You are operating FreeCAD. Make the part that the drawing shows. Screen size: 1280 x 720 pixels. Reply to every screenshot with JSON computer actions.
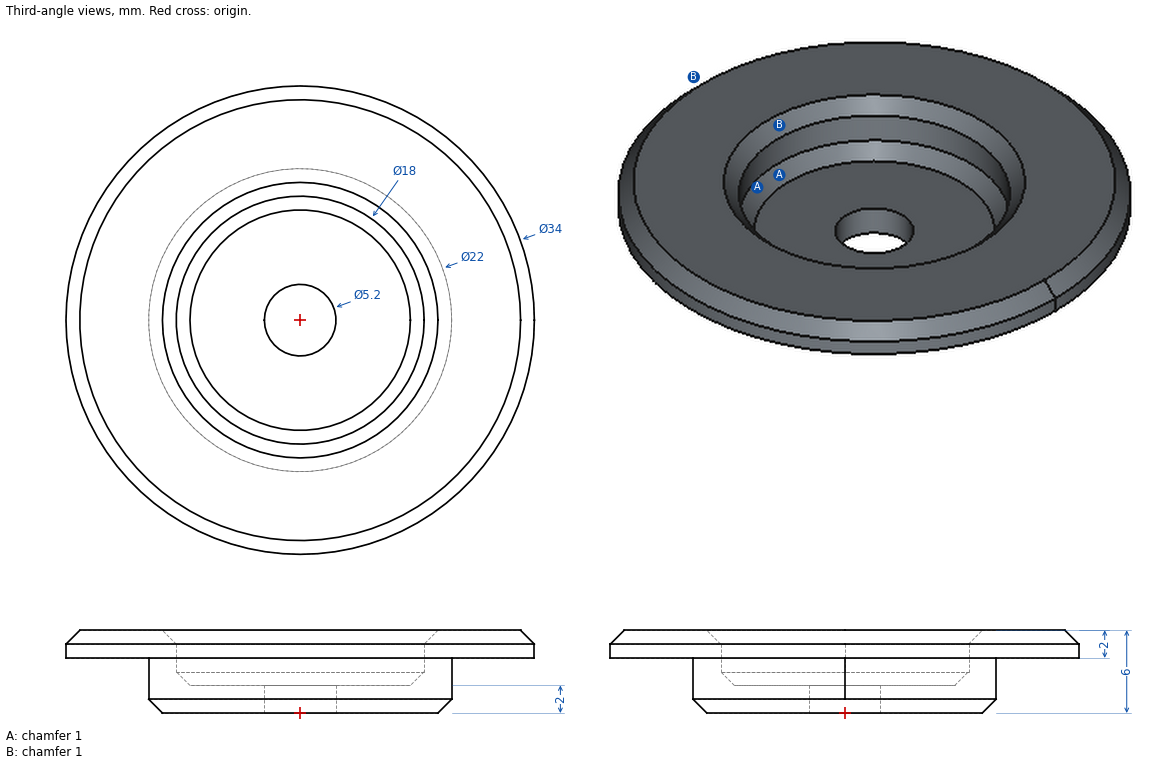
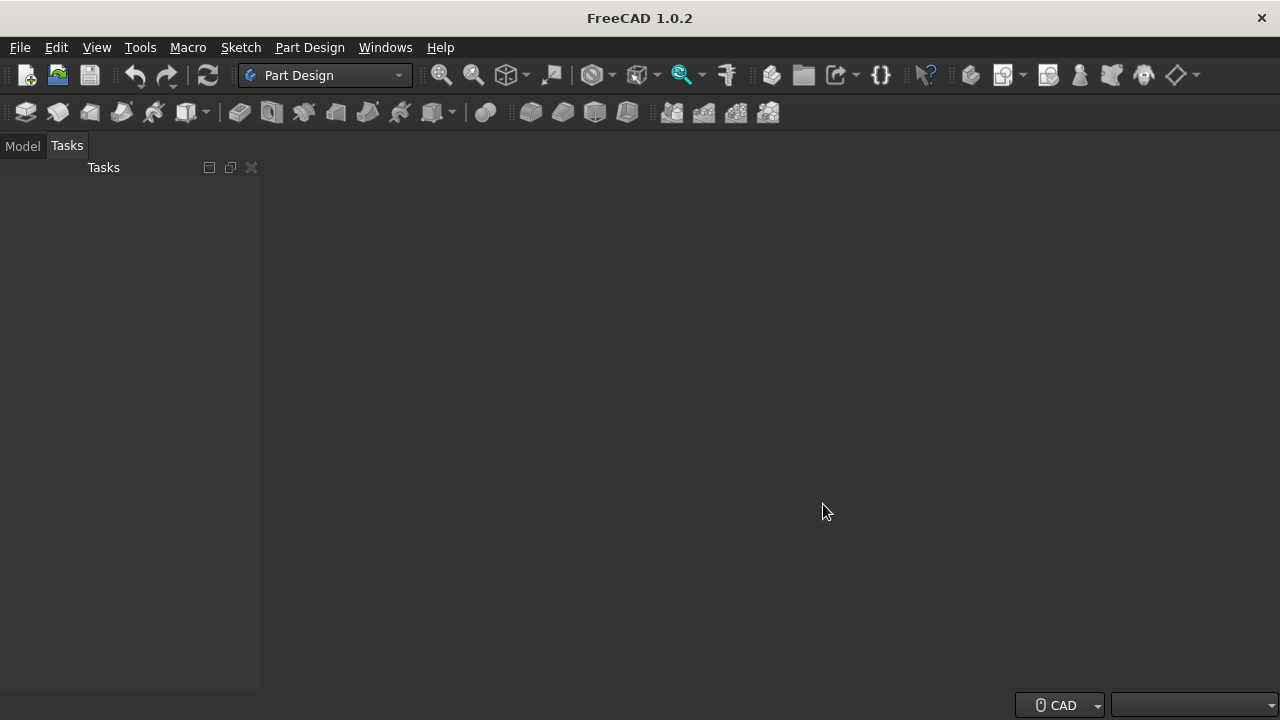
{"action": "left_click", "coordinate": [26, 76]}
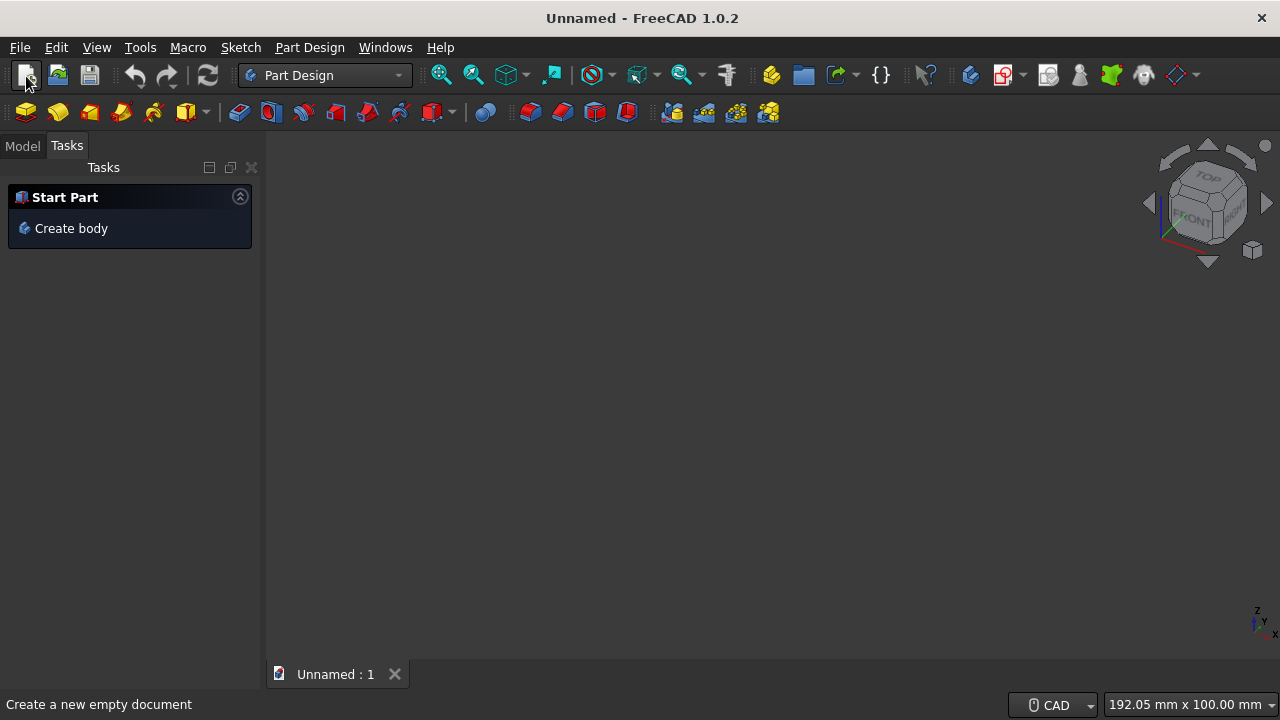
{"action": "left_click", "coordinate": [1004, 76]}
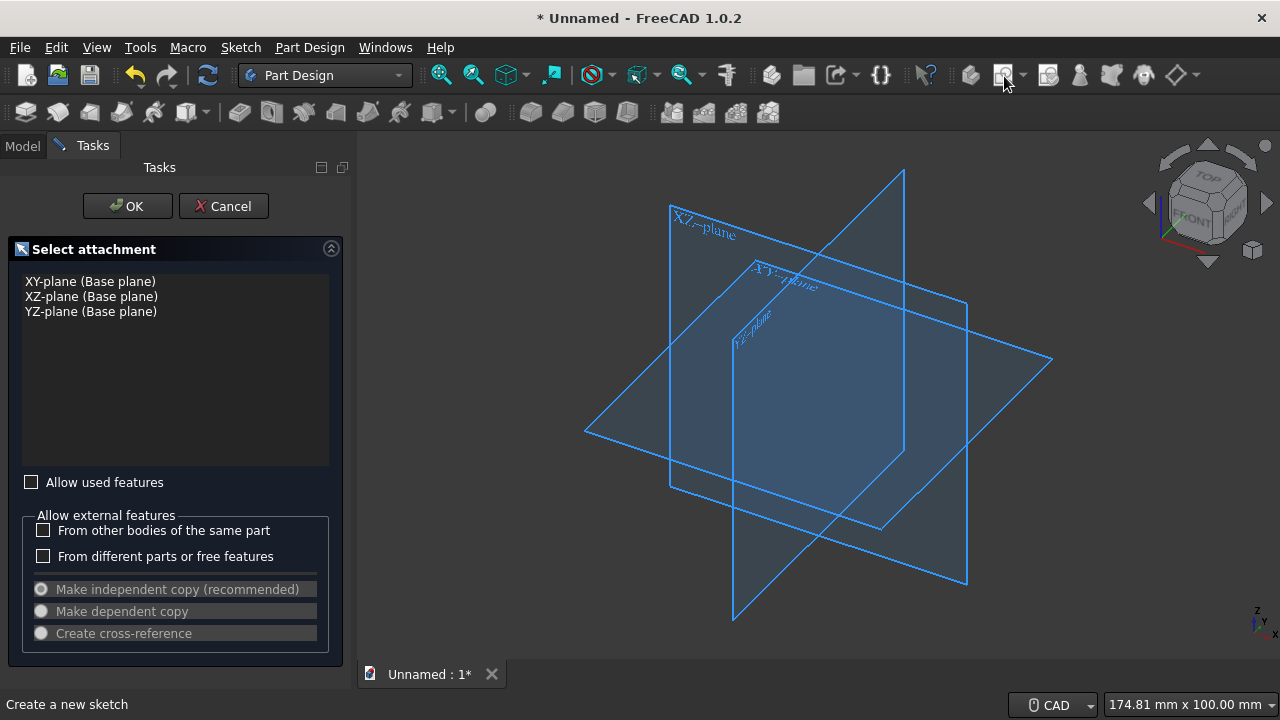
{"action": "left_click", "coordinate": [82, 282]}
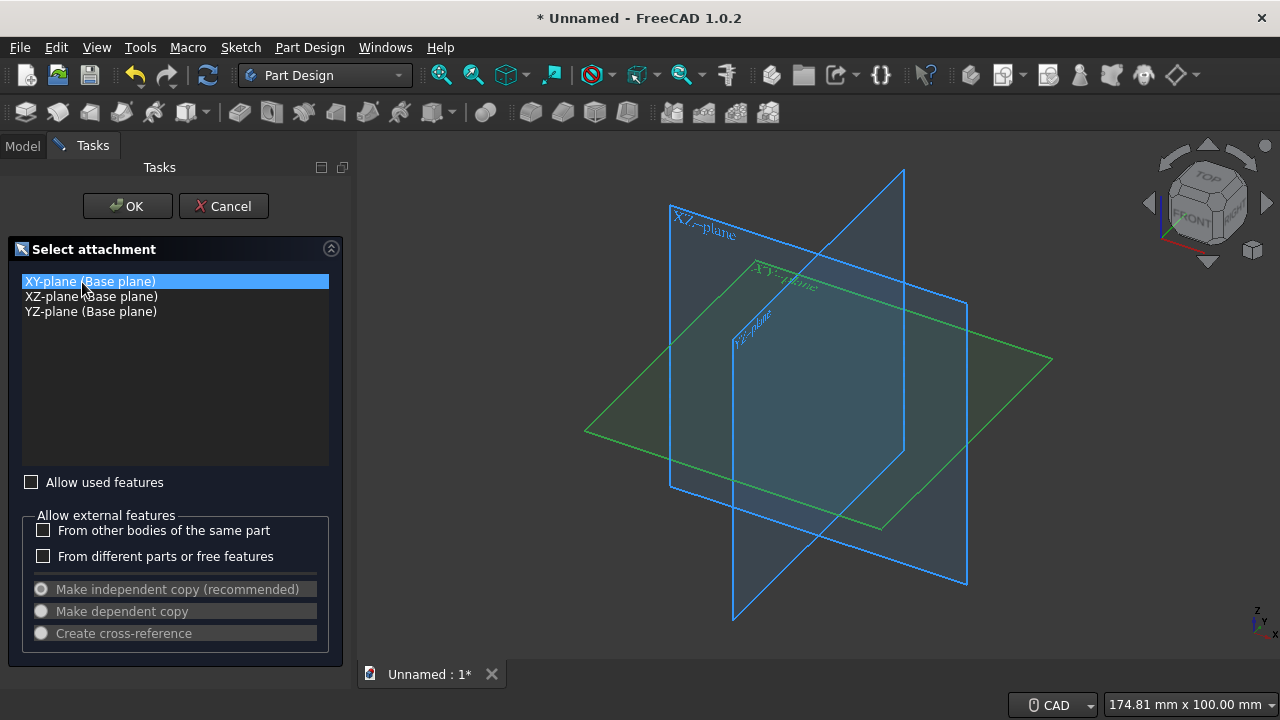
{"action": "left_click", "coordinate": [128, 206]}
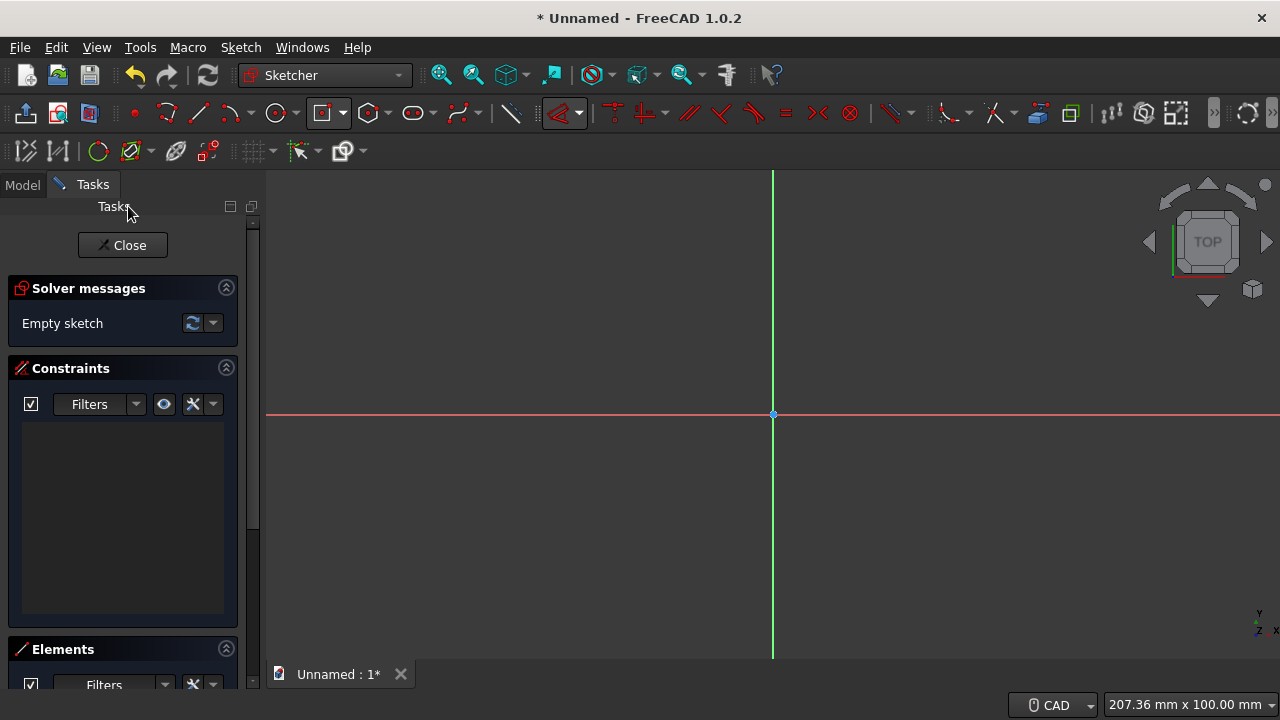
{"action": "scroll", "coordinate": [813, 415], "scroll_direction": "up", "scroll_amount": 5}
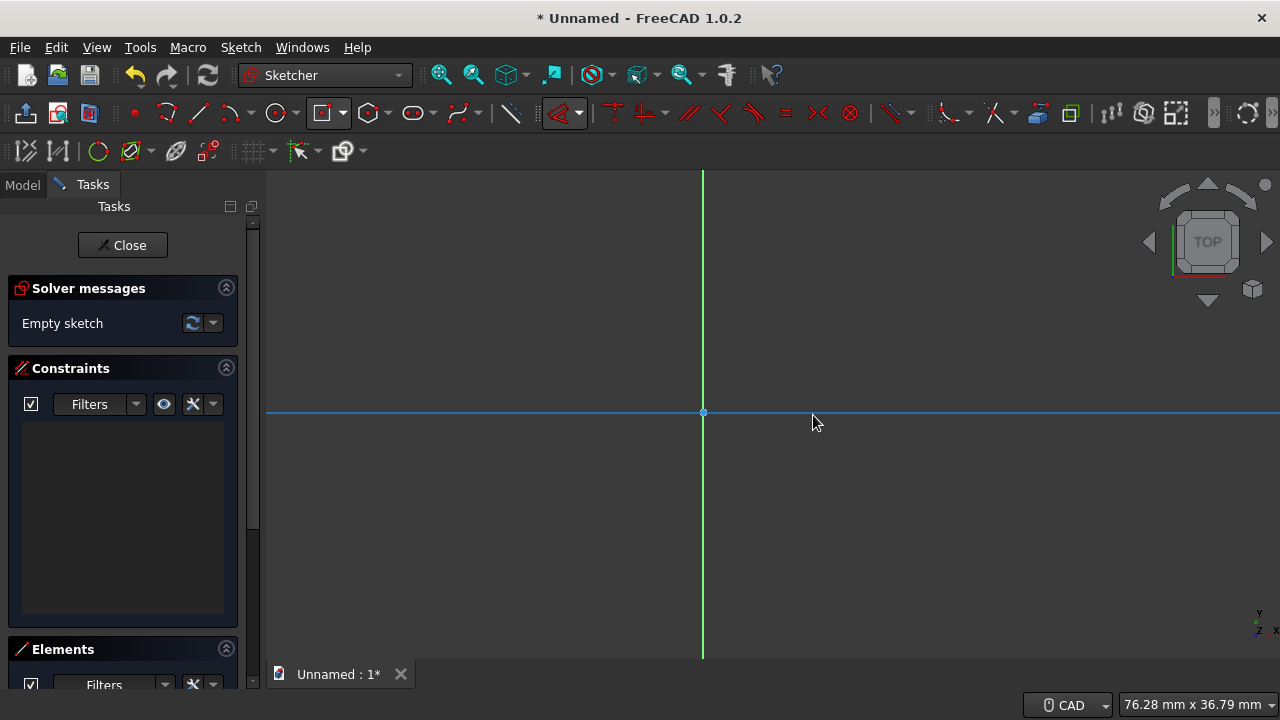
{"action": "left_click", "coordinate": [276, 114]}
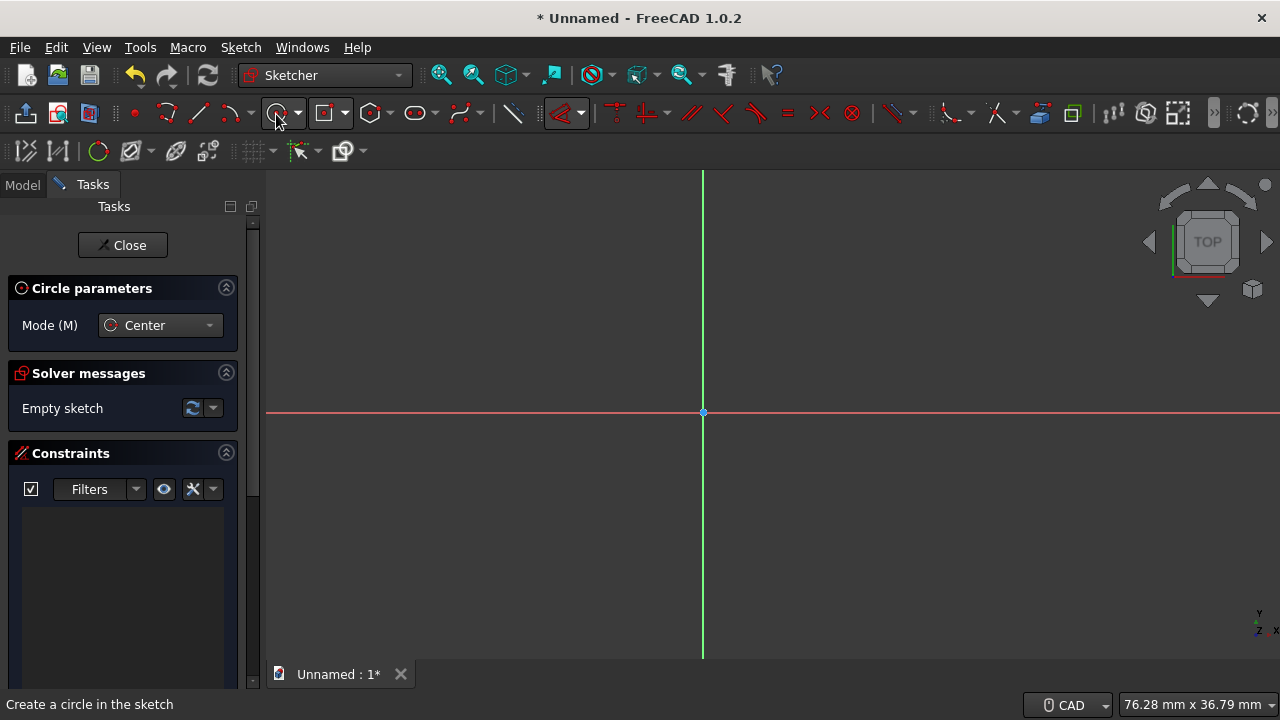
{"action": "left_click", "coordinate": [703, 413]}
{"action": "mouse_move", "coordinate": [807, 309]}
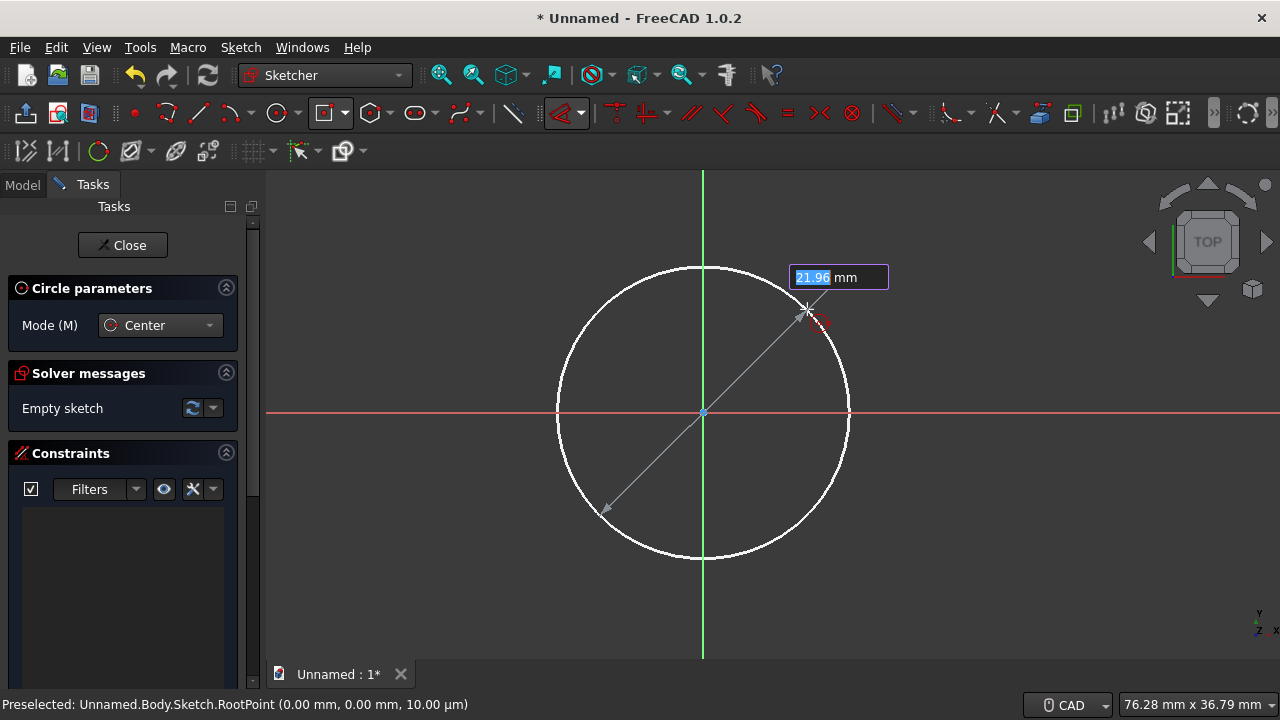
{"action": "type", "text": "22"}
{"action": "key", "text": "Return"}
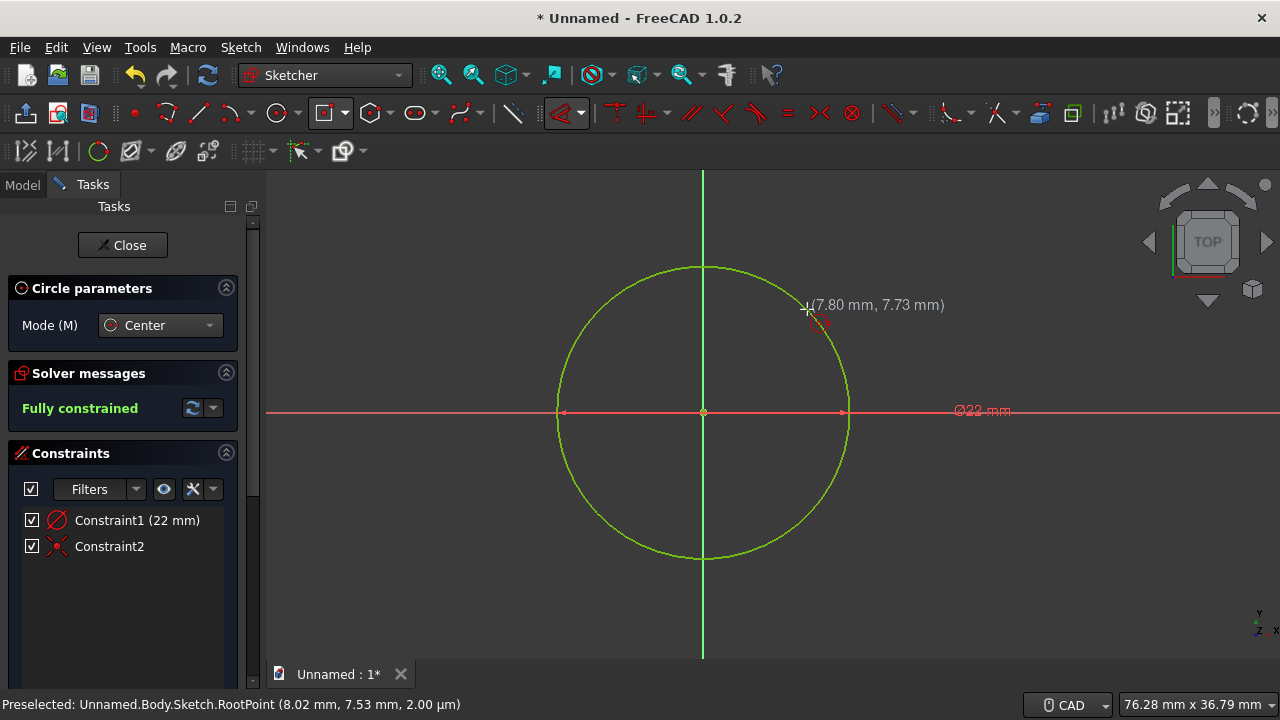
{"action": "left_click", "coordinate": [703, 413]}
{"action": "mouse_move", "coordinate": [788, 328]}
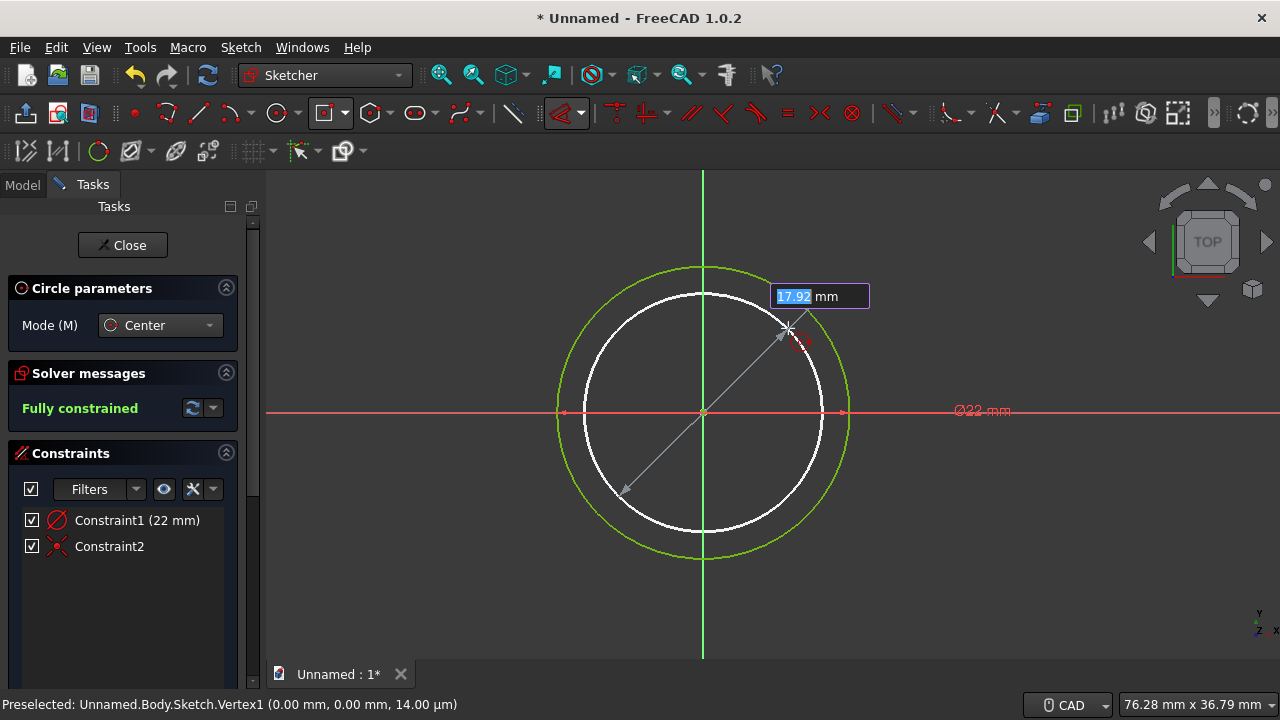
{"action": "type", "text": "18"}
{"action": "key", "text": "Return"}
{"action": "key", "text": "Escape"}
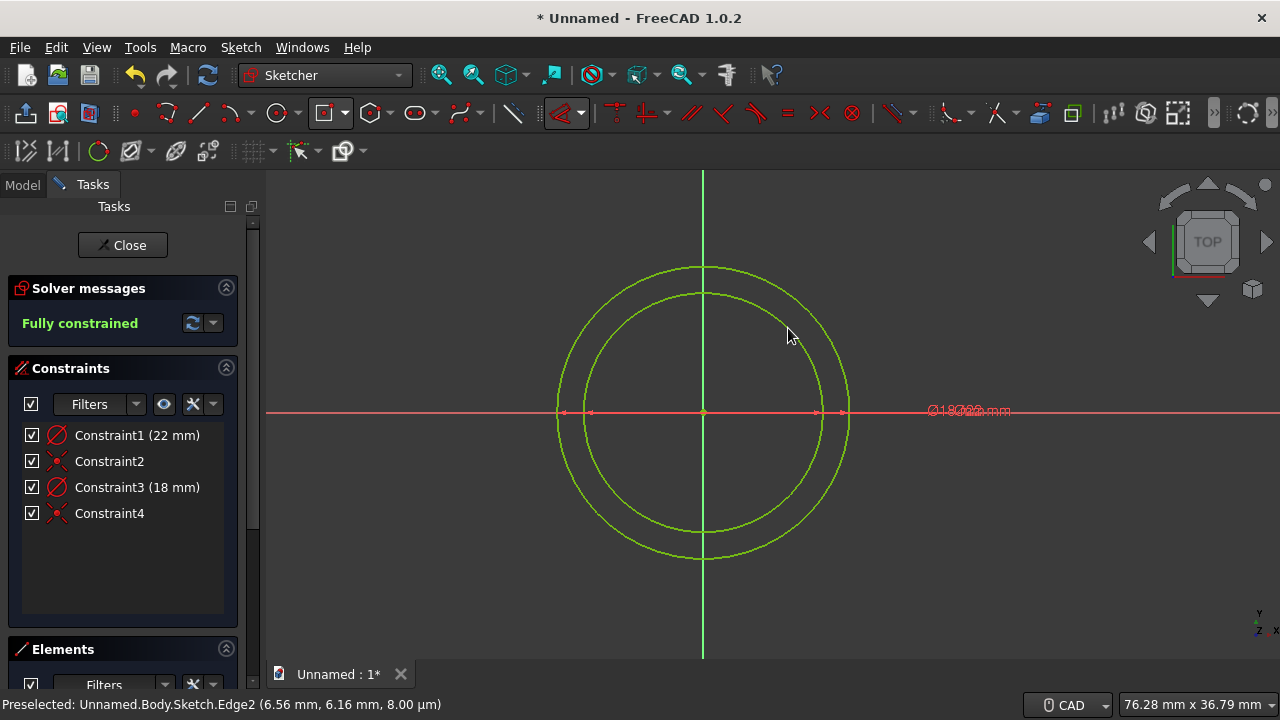
{"action": "left_click", "coordinate": [123, 245]}